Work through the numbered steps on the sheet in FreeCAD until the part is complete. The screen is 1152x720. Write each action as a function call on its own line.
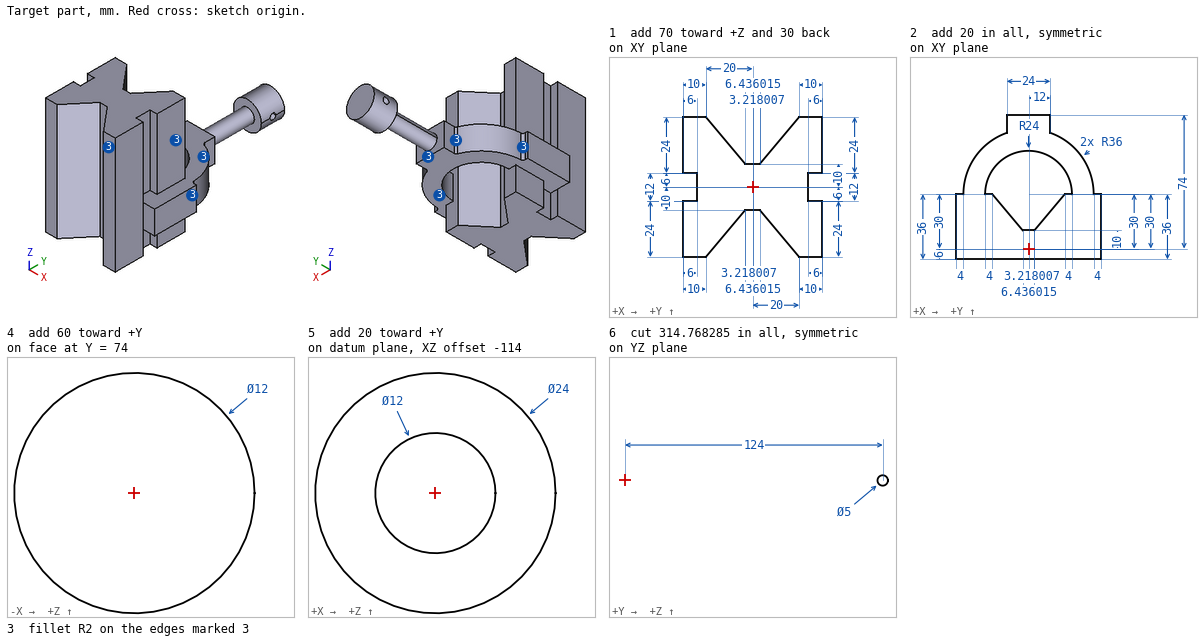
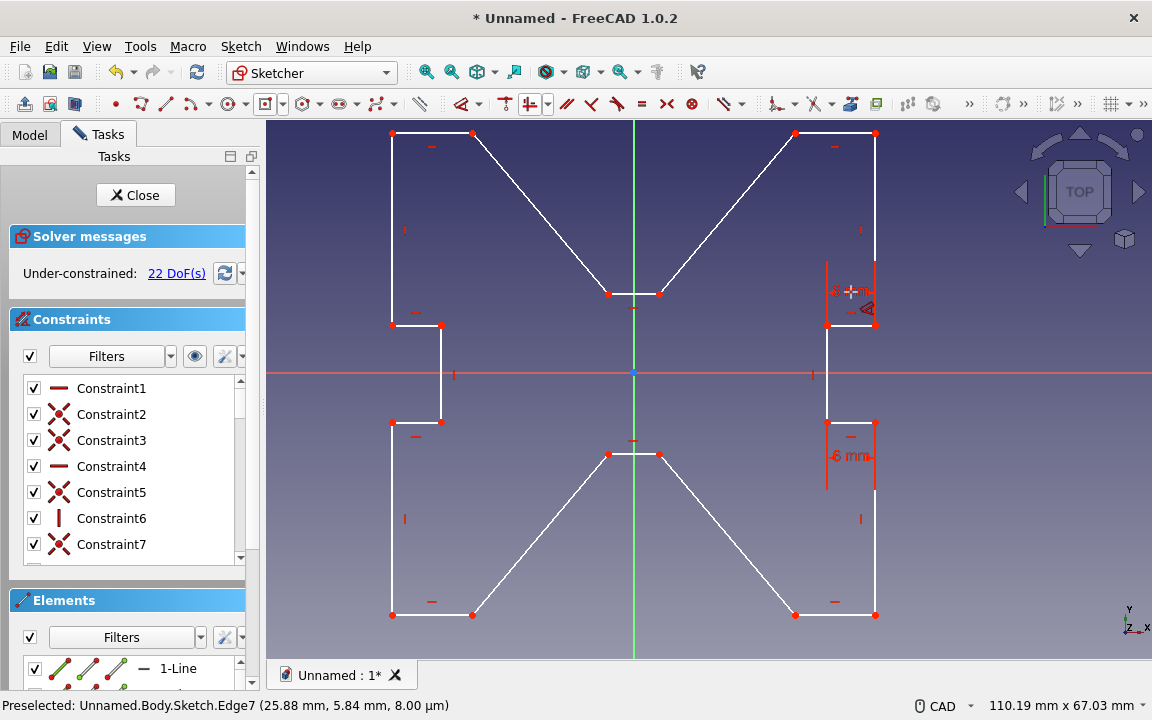
click(407, 326)
click(417, 292)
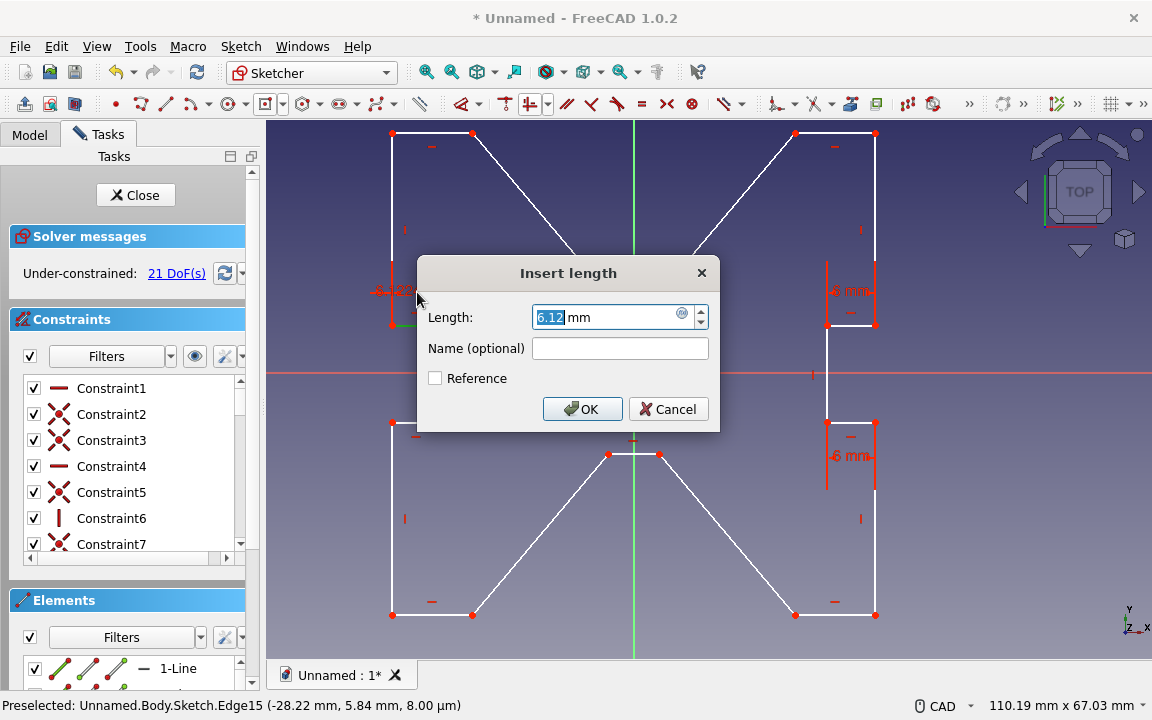
text(6)
key(Return)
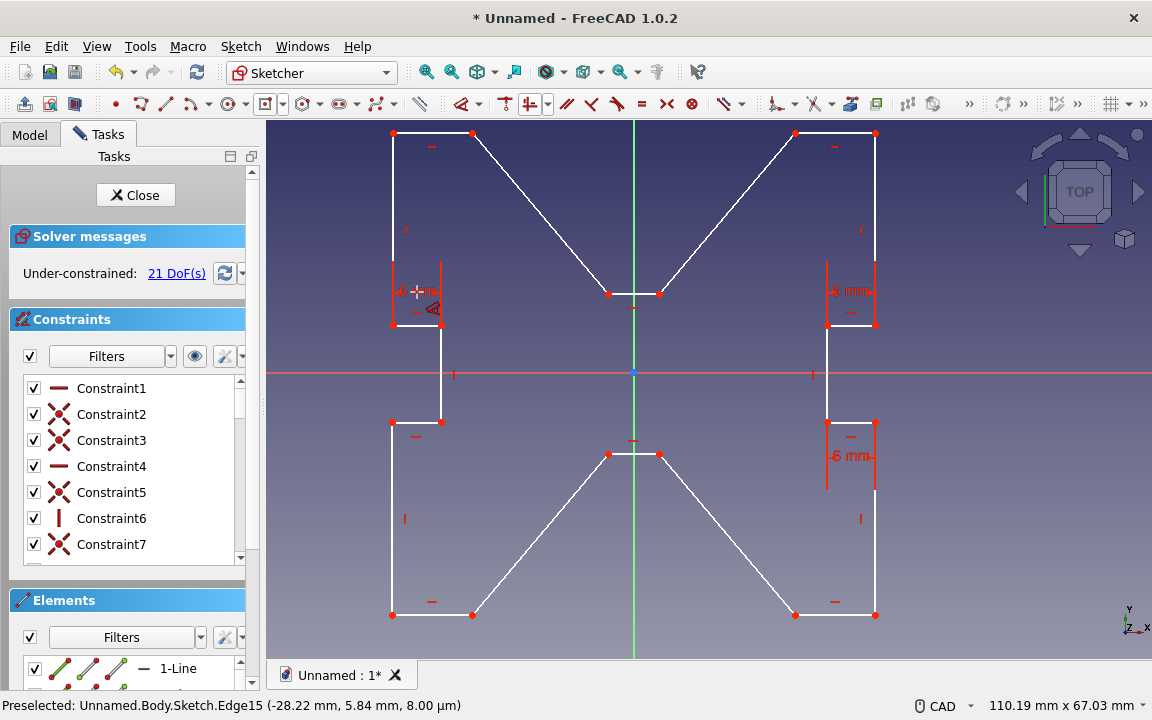
click(427, 423)
click(417, 457)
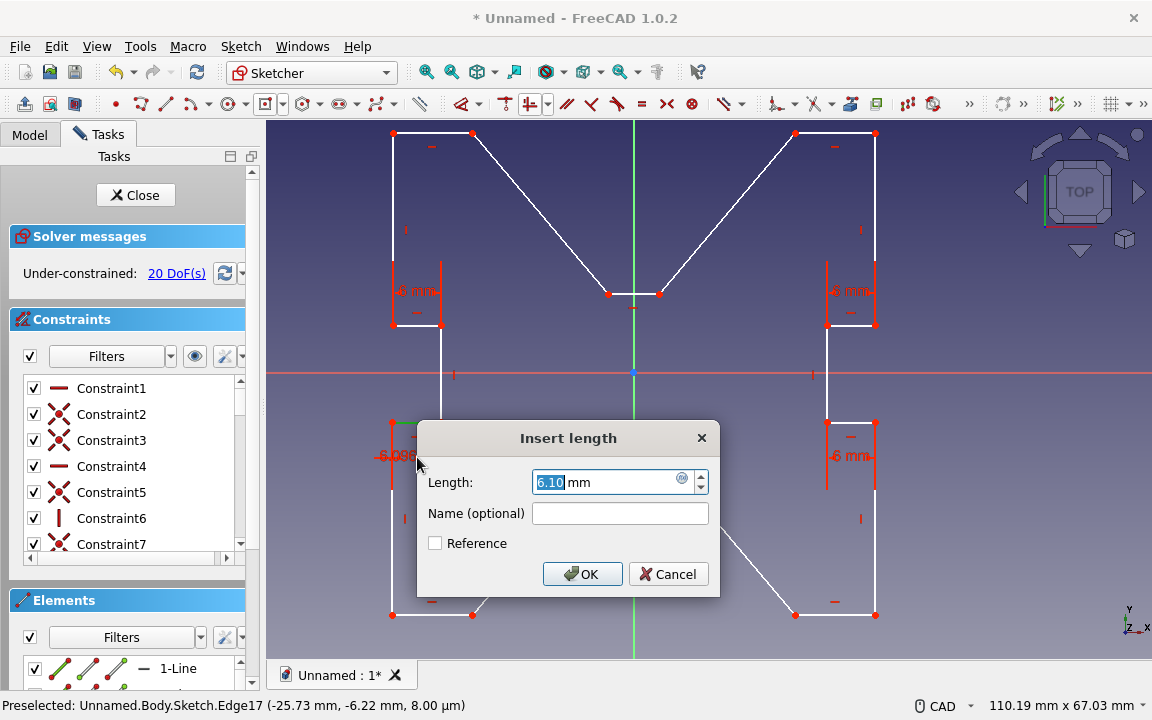
text(6)
key(Return)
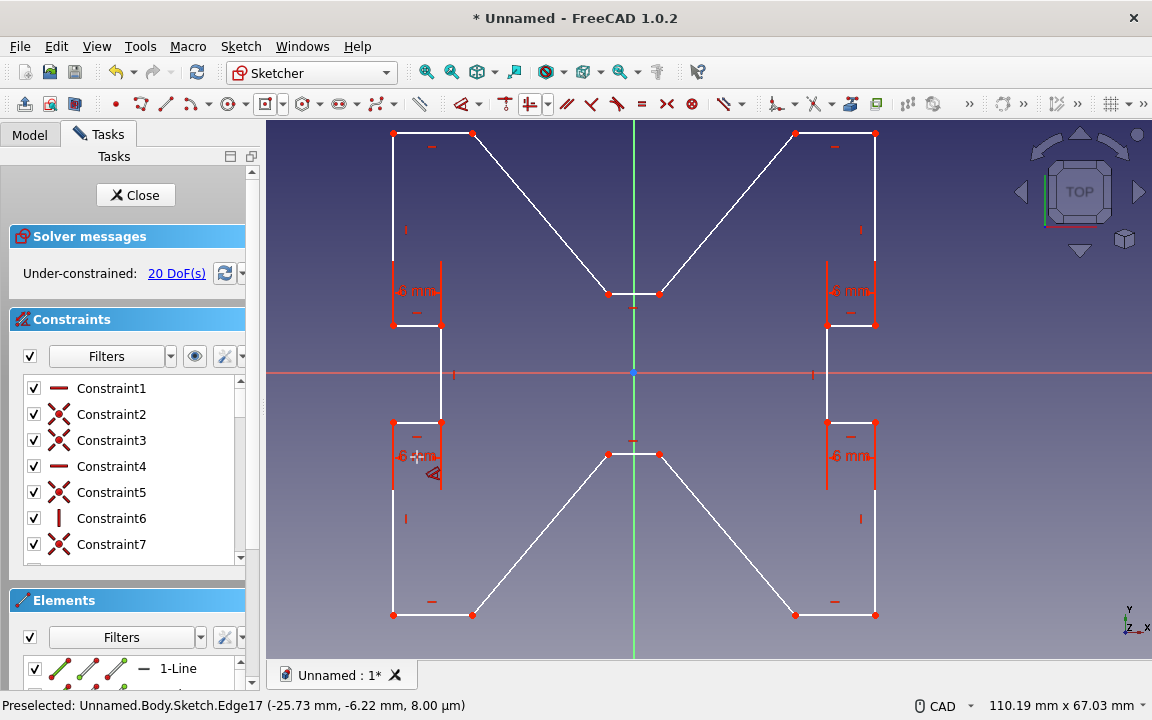
click(819, 615)
click(835, 581)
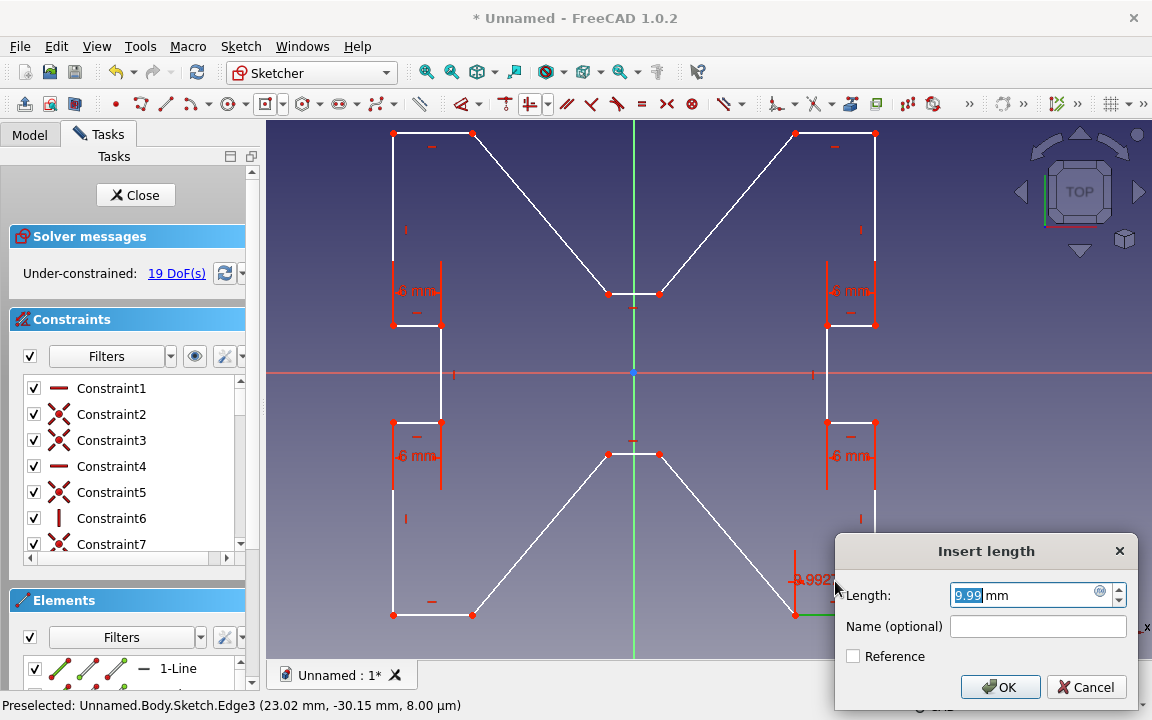
text(10)
key(Return)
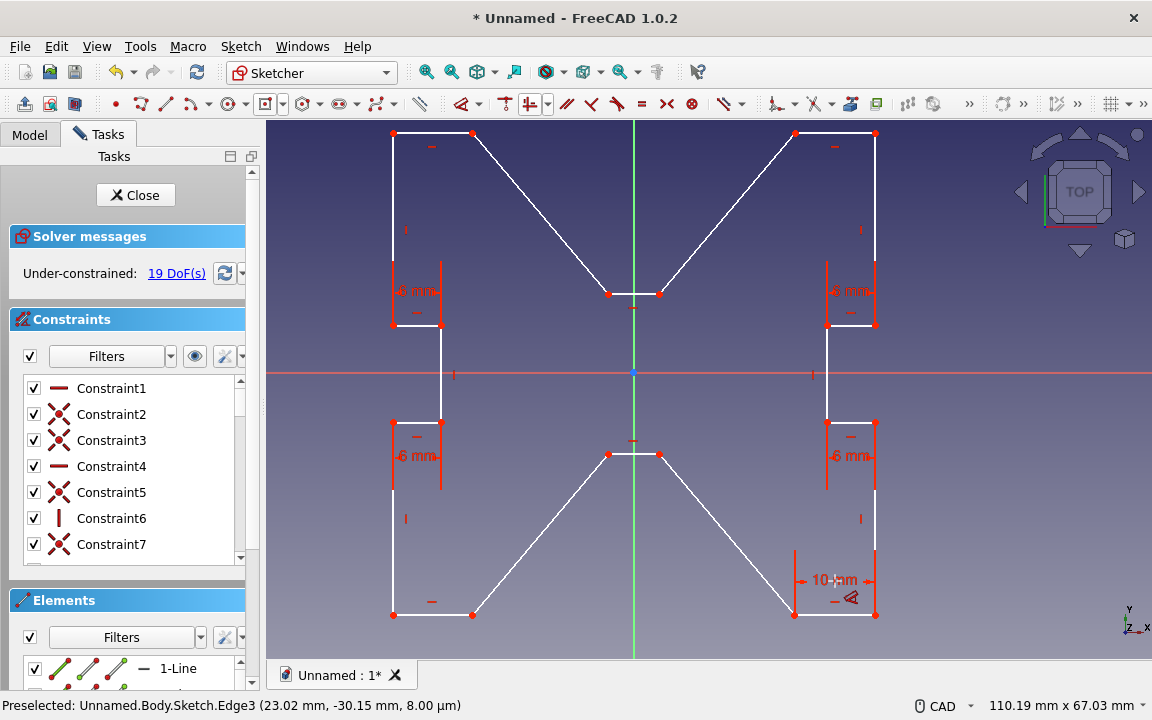
click(875, 557)
click(909, 519)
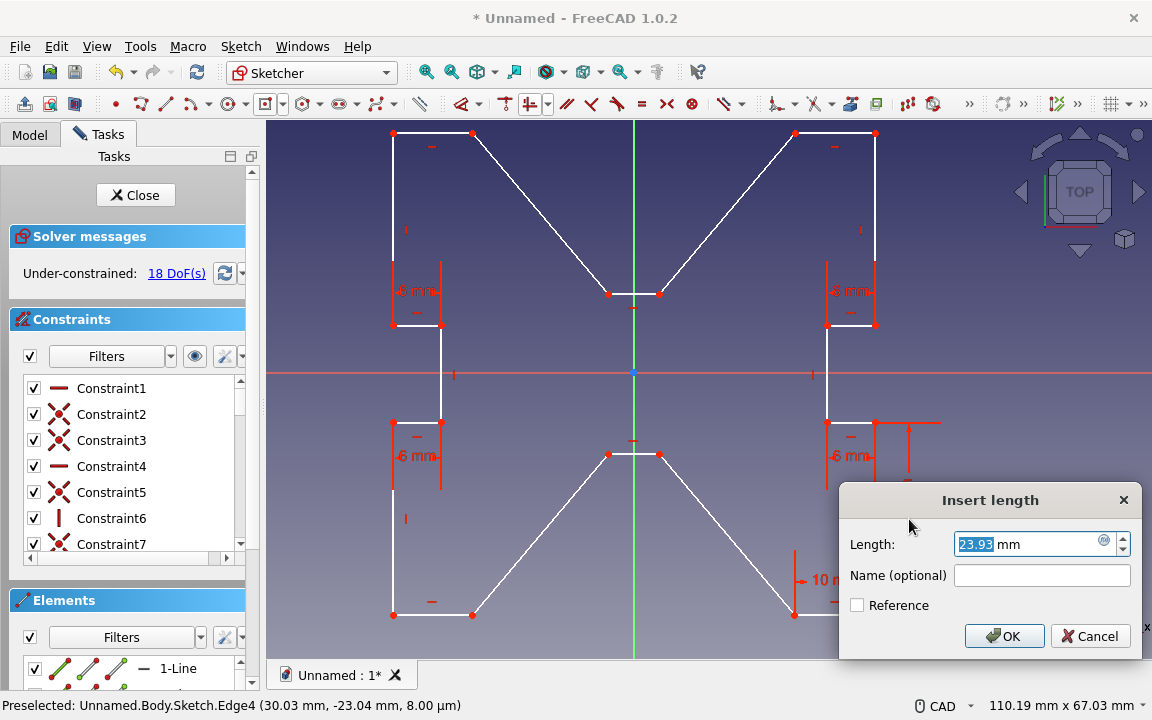
text(24)
key(Return)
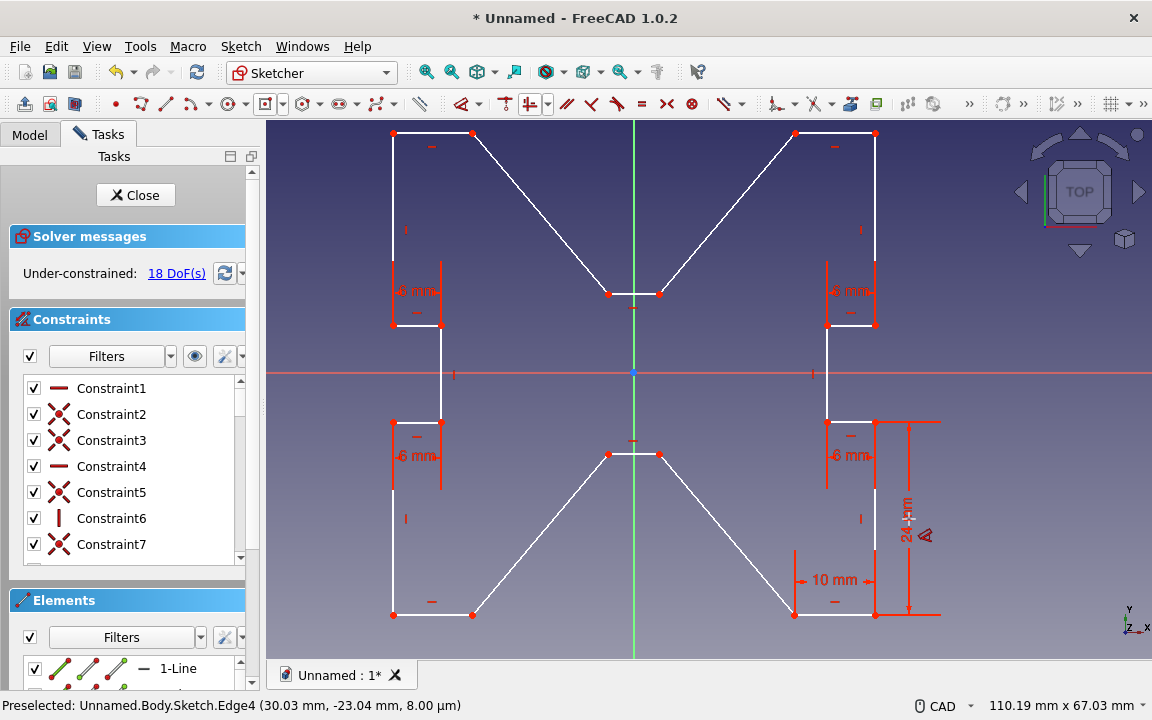
click(827, 393)
click(861, 352)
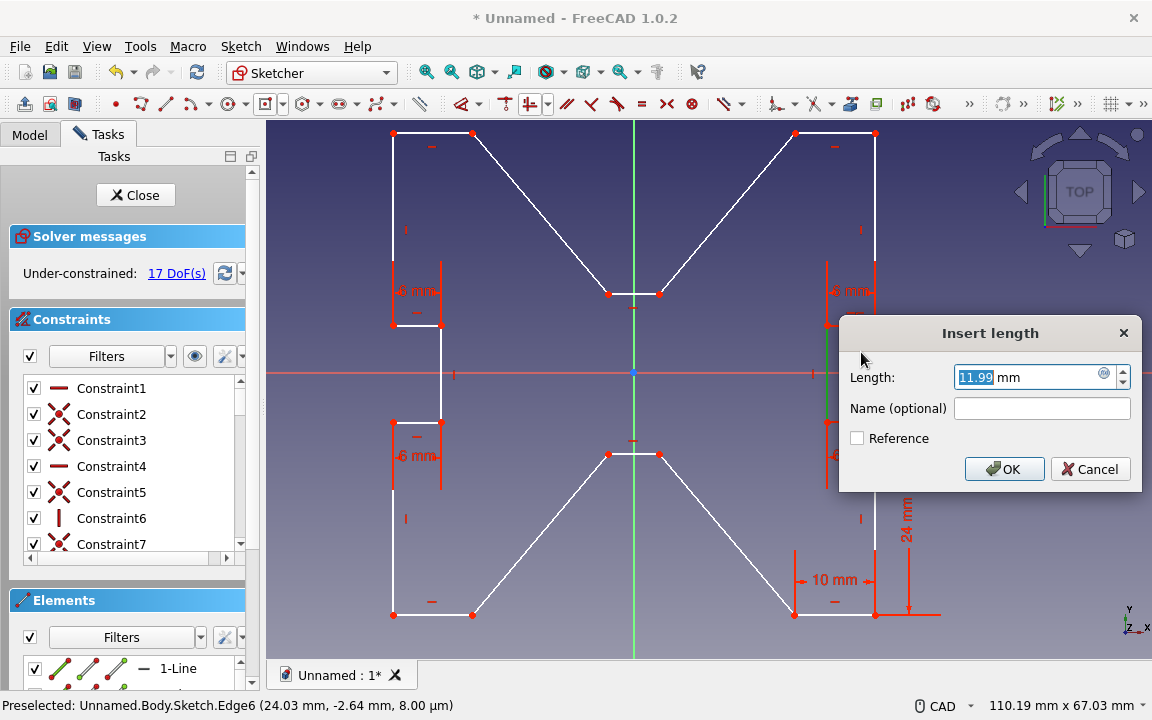
text(12)
key(Return)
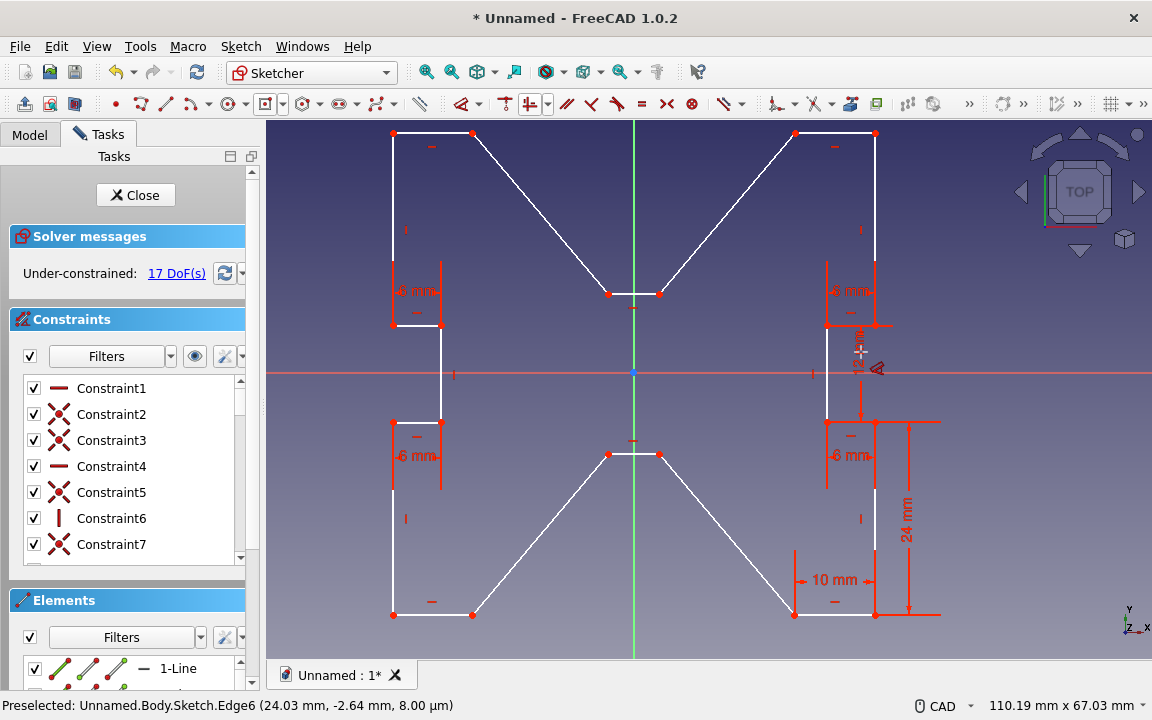
click(875, 268)
click(909, 237)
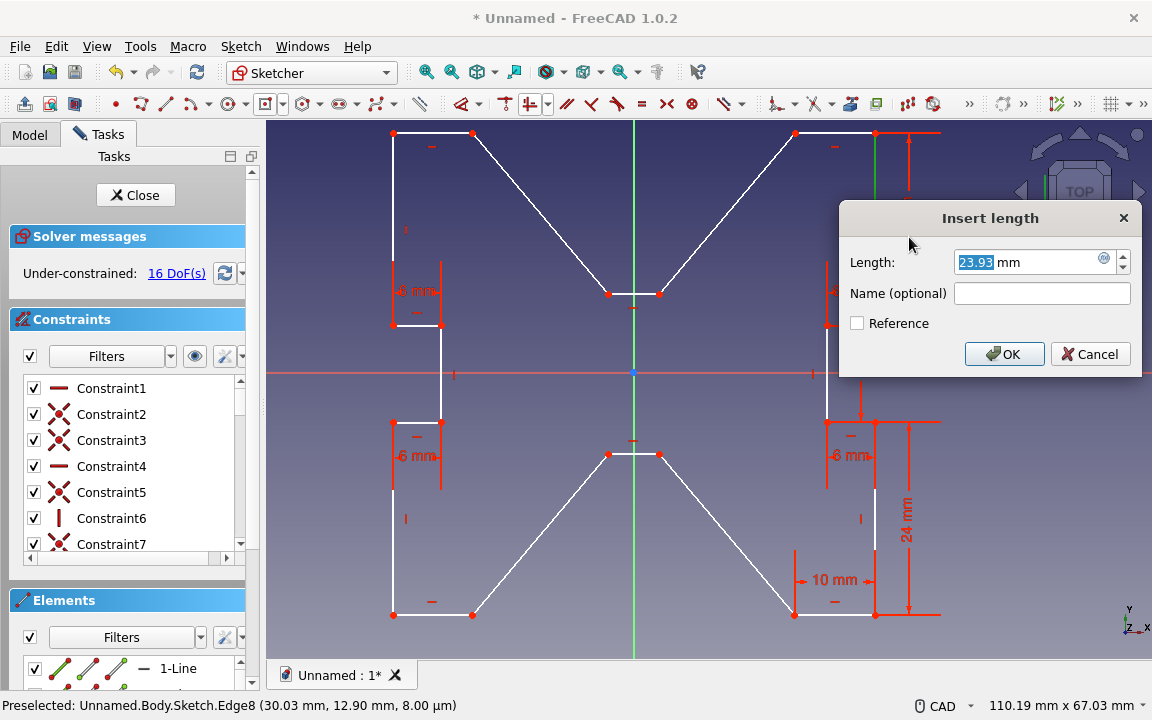
text(24)
key(Return)